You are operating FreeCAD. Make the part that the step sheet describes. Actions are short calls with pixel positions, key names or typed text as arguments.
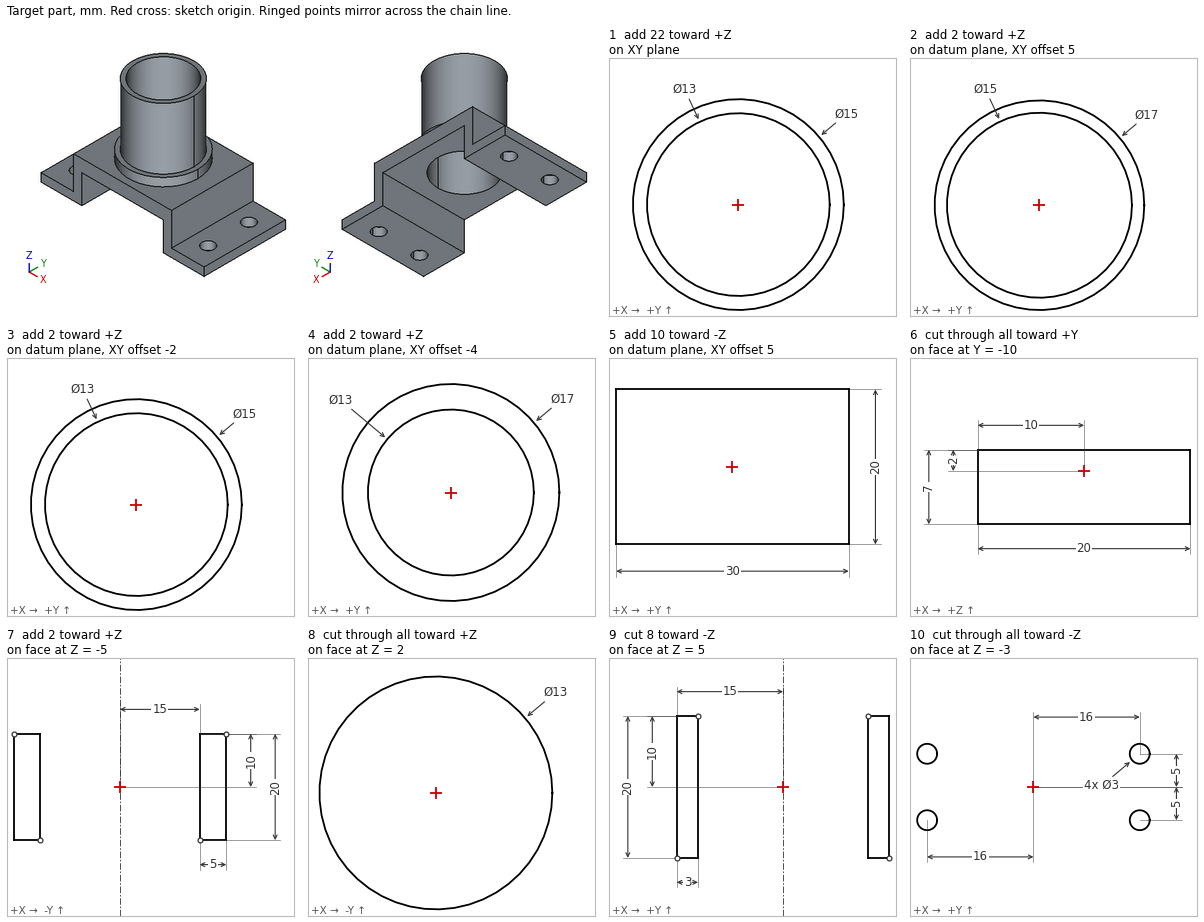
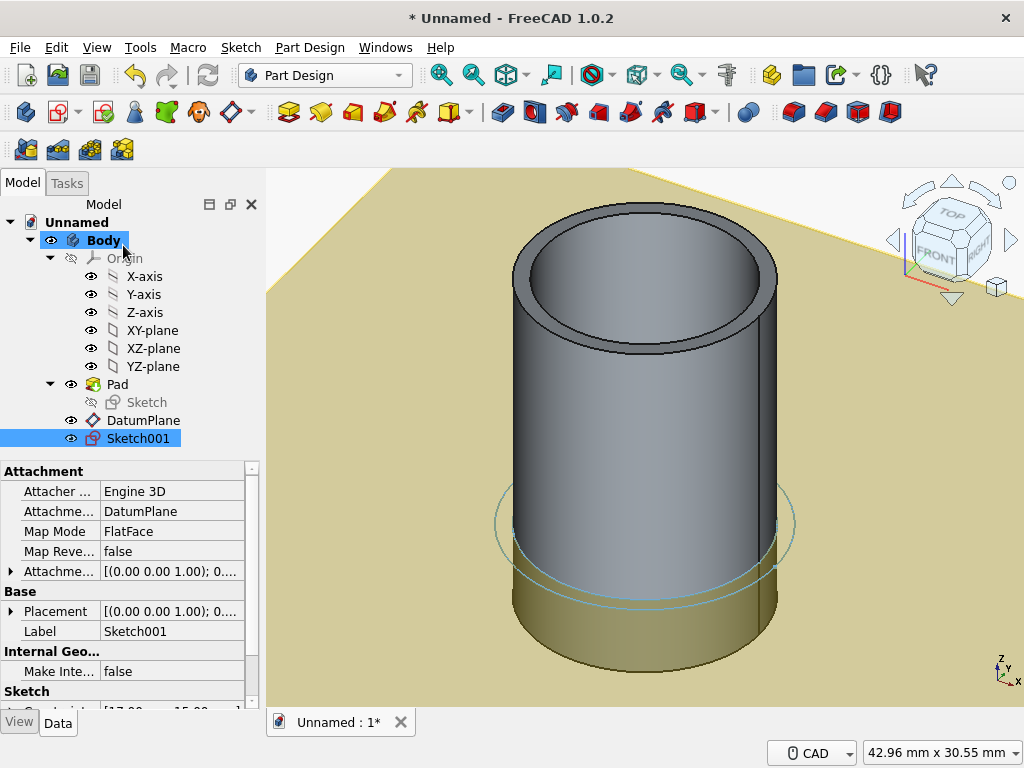
click(290, 112)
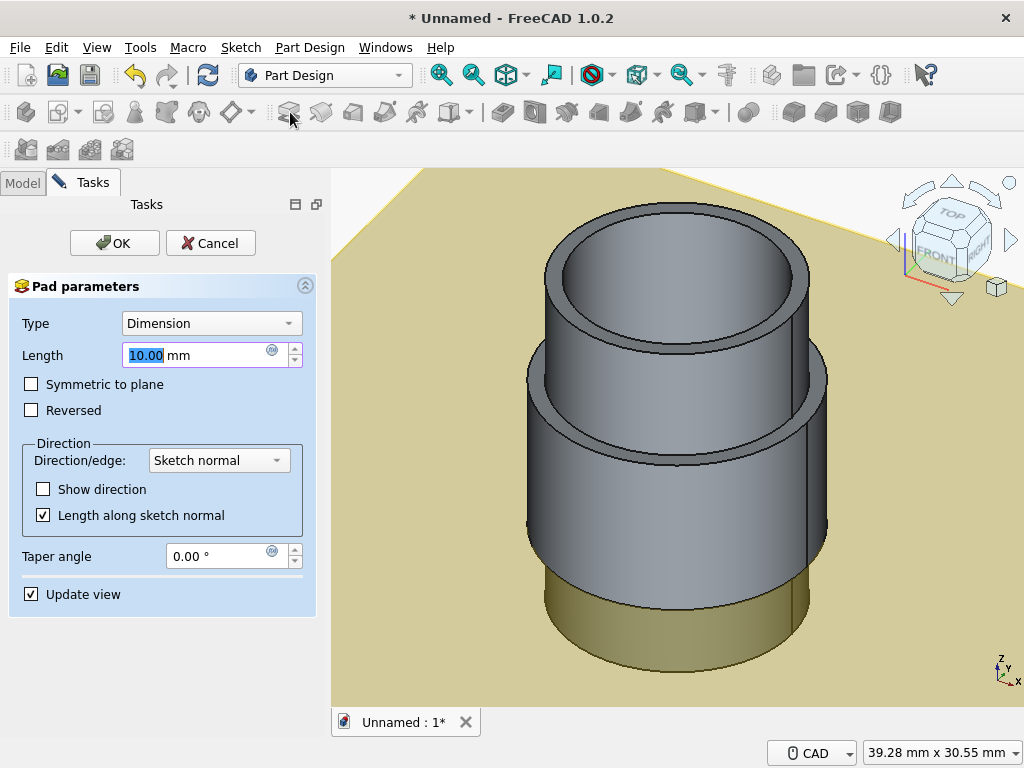
text(2)
key(Tab)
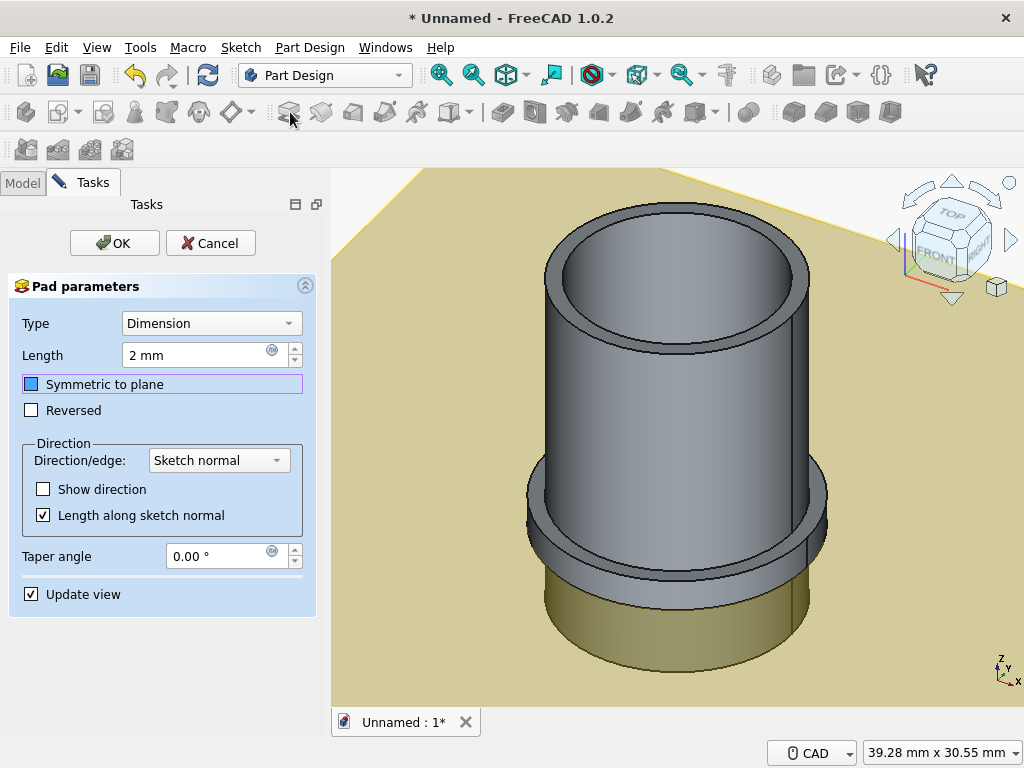
click(115, 243)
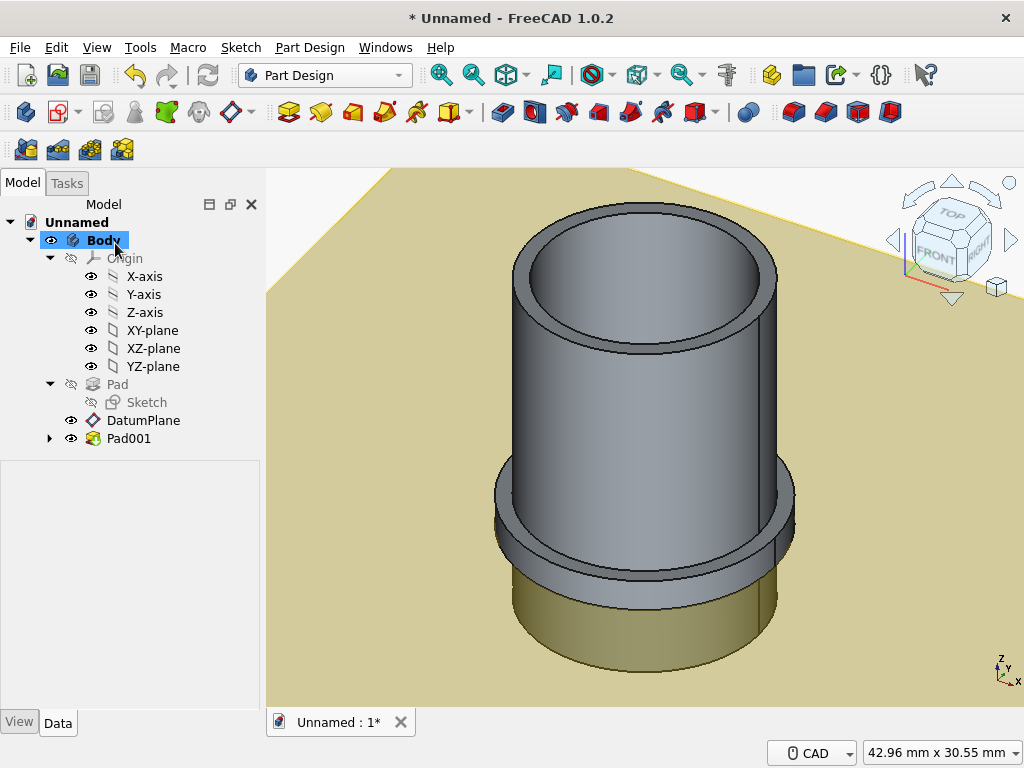
click(116, 420)
key(space)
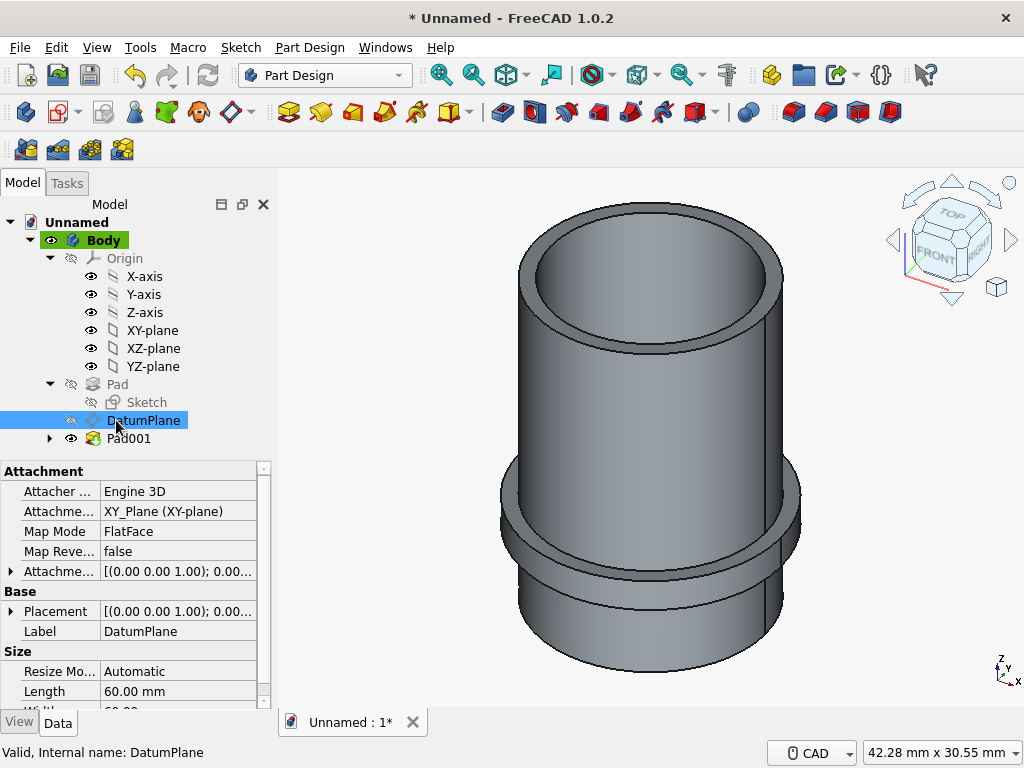
key(v)
key(f)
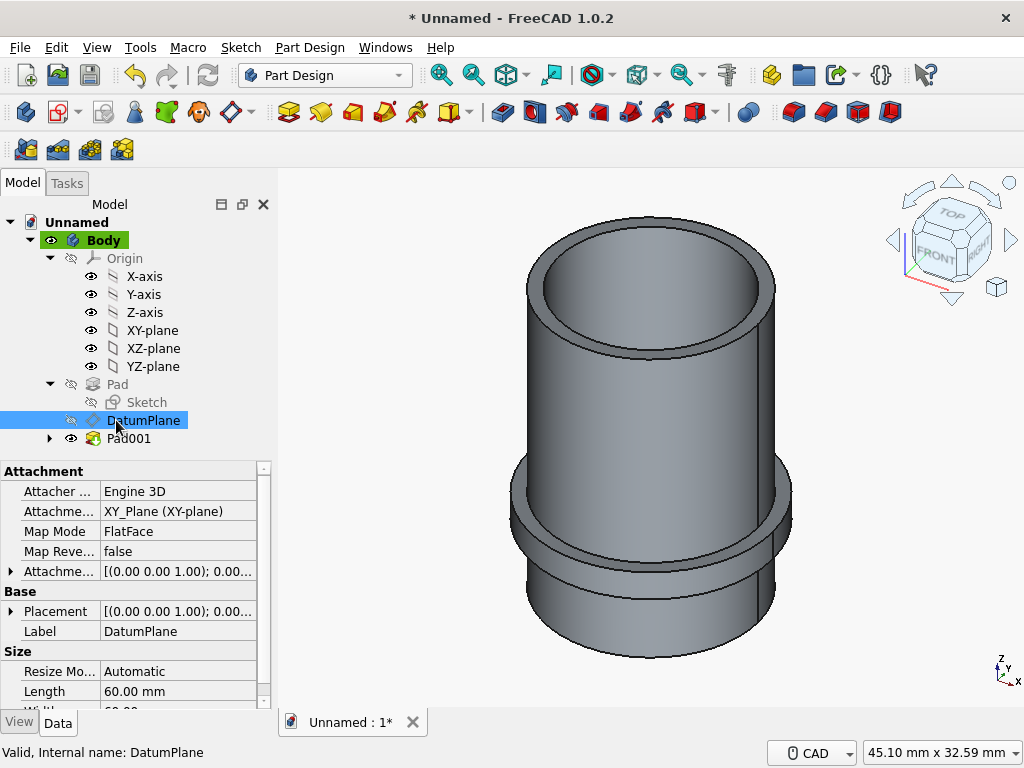
click(136, 330)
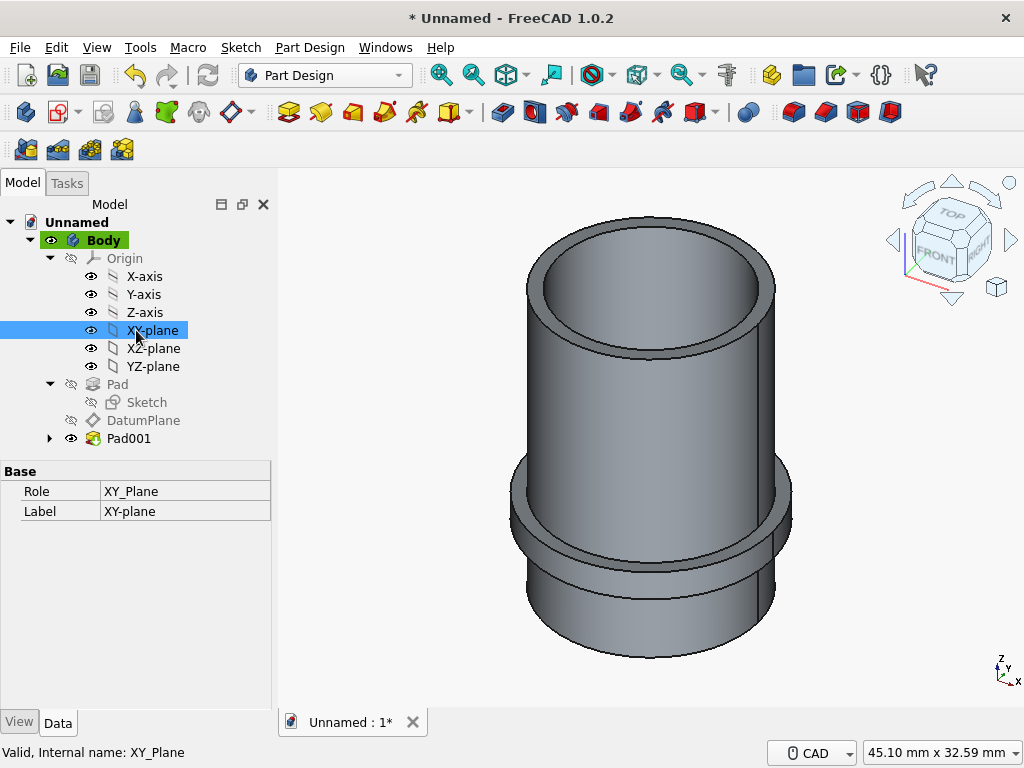
click(232, 112)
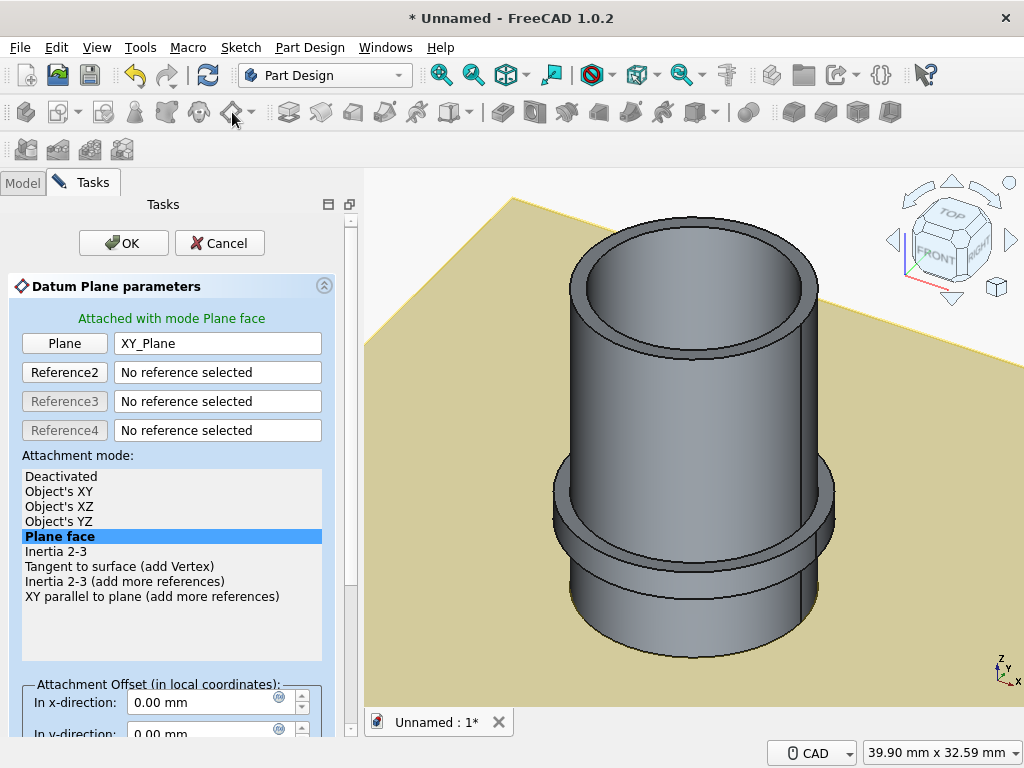
scroll(351, 475, down, 2)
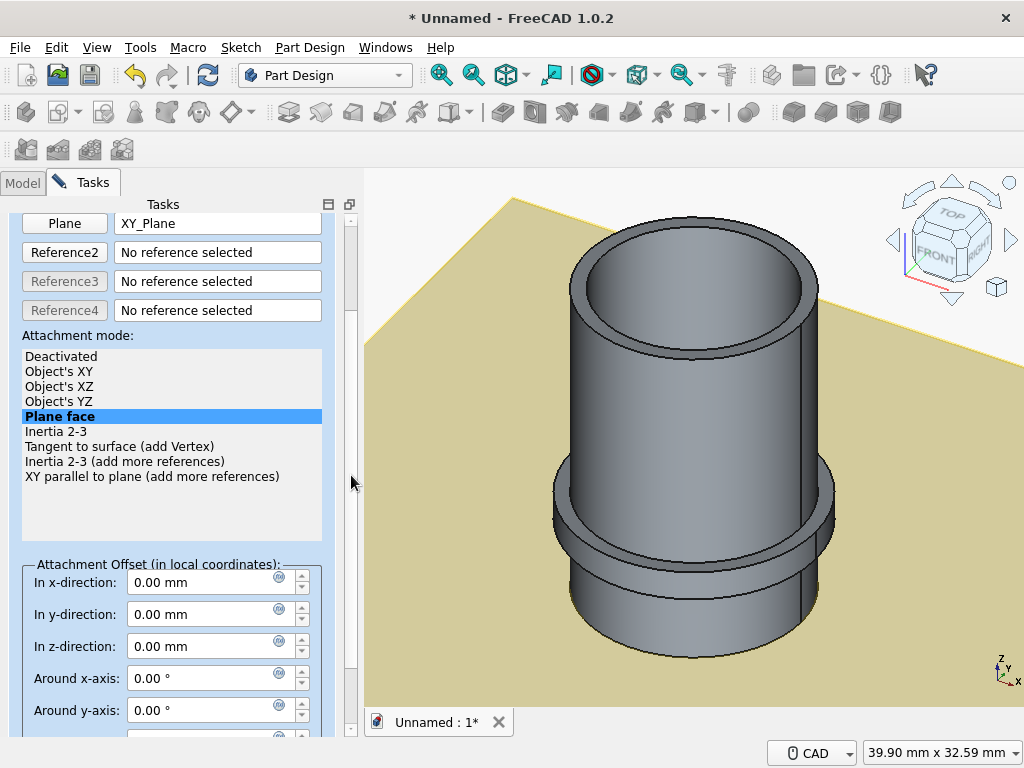
triple_click(210, 646)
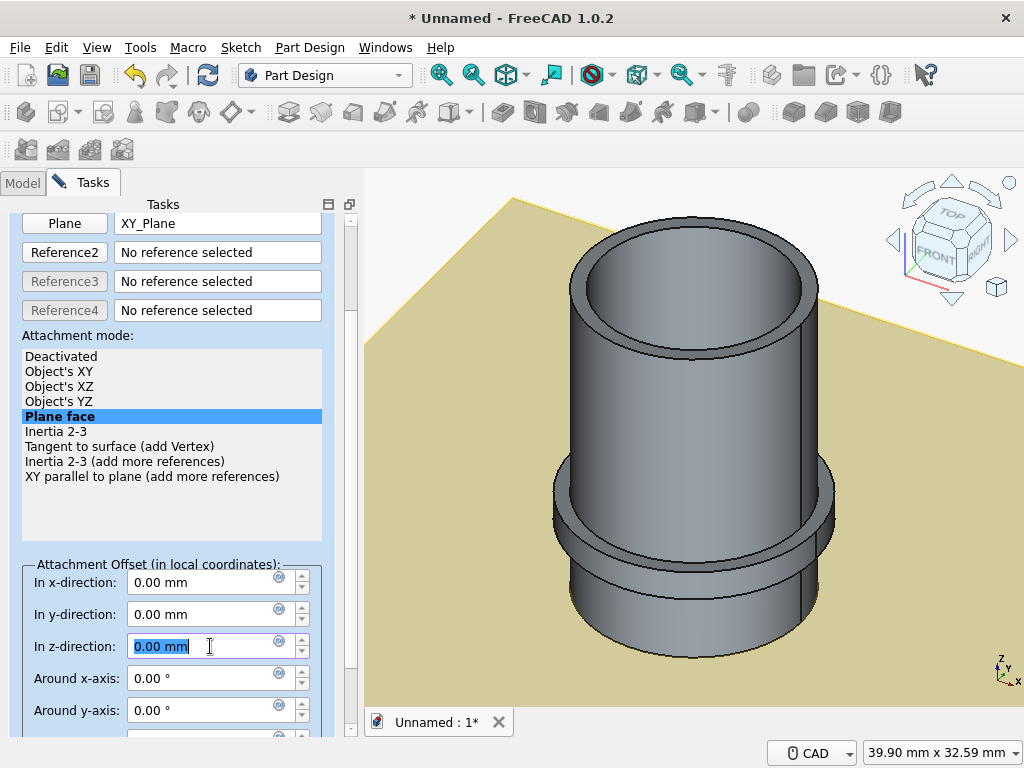
text(-2)
key(Tab)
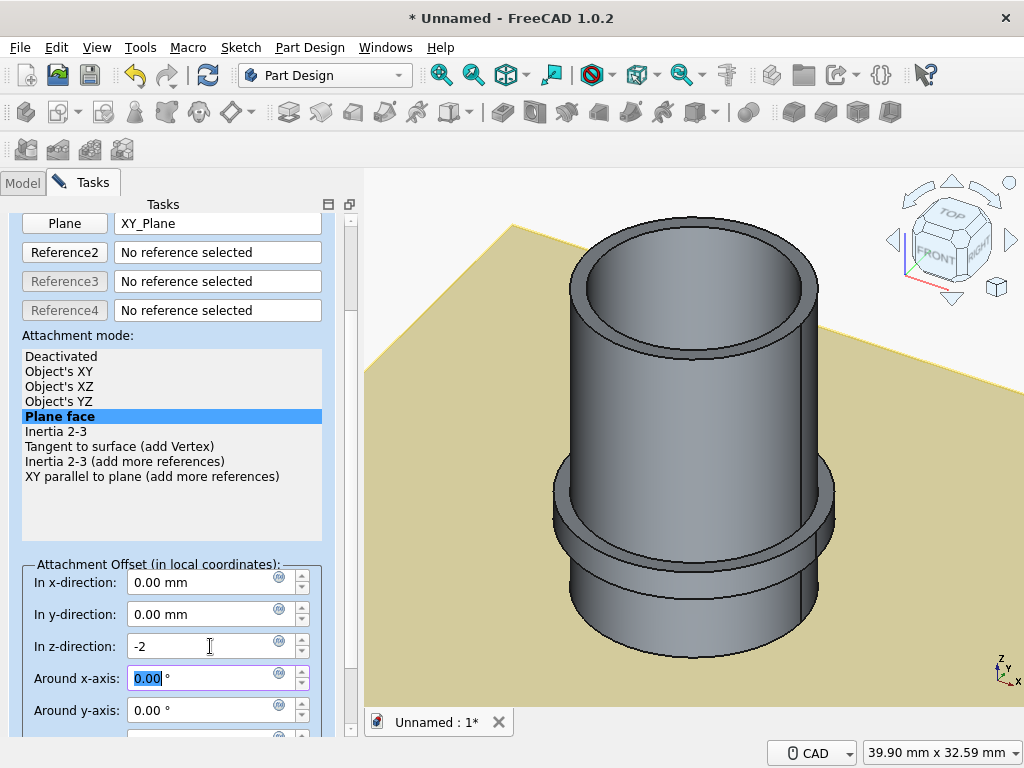
scroll(351, 475, up, 3)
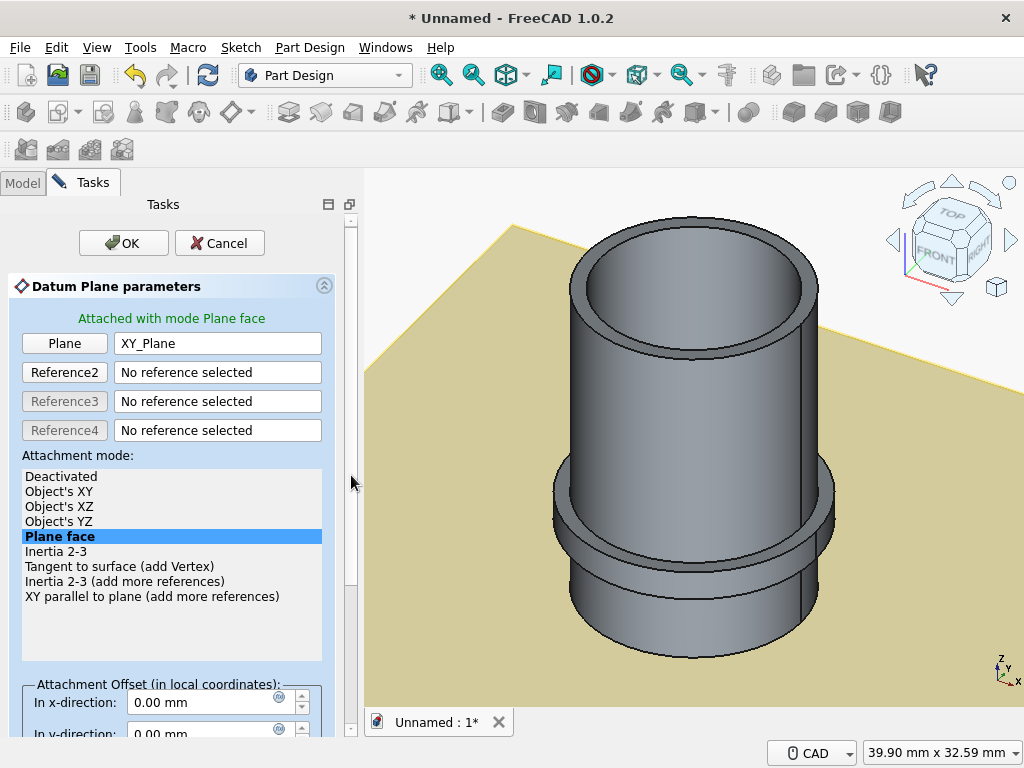
click(124, 243)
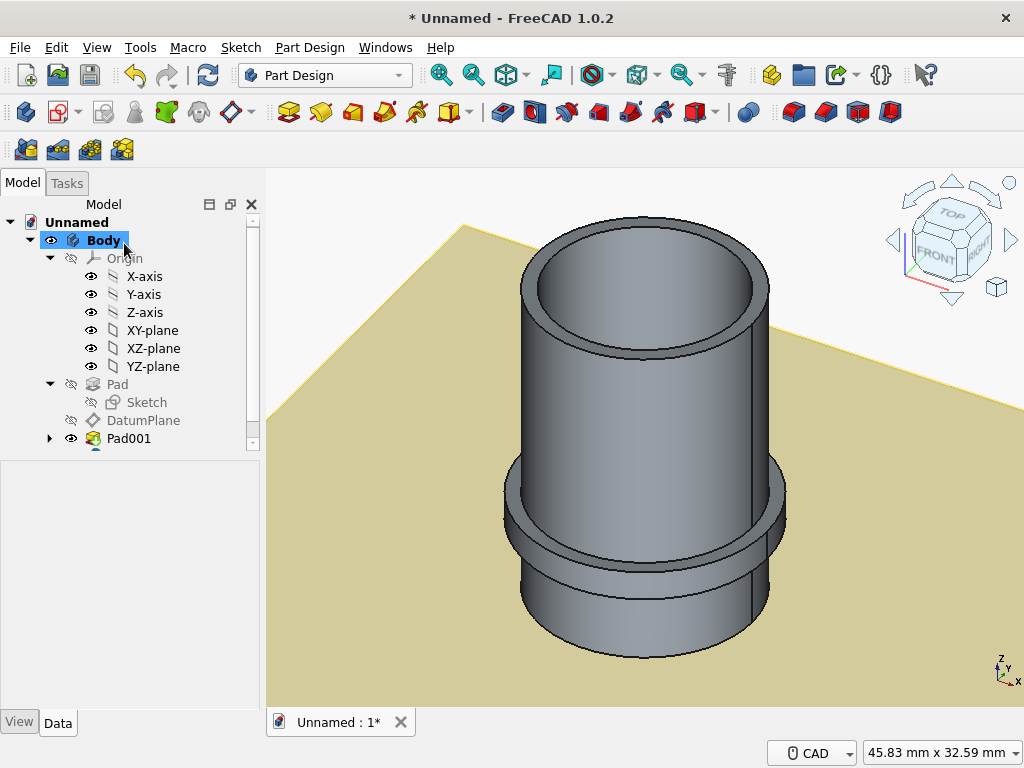
scroll(100, 326, down, 3)